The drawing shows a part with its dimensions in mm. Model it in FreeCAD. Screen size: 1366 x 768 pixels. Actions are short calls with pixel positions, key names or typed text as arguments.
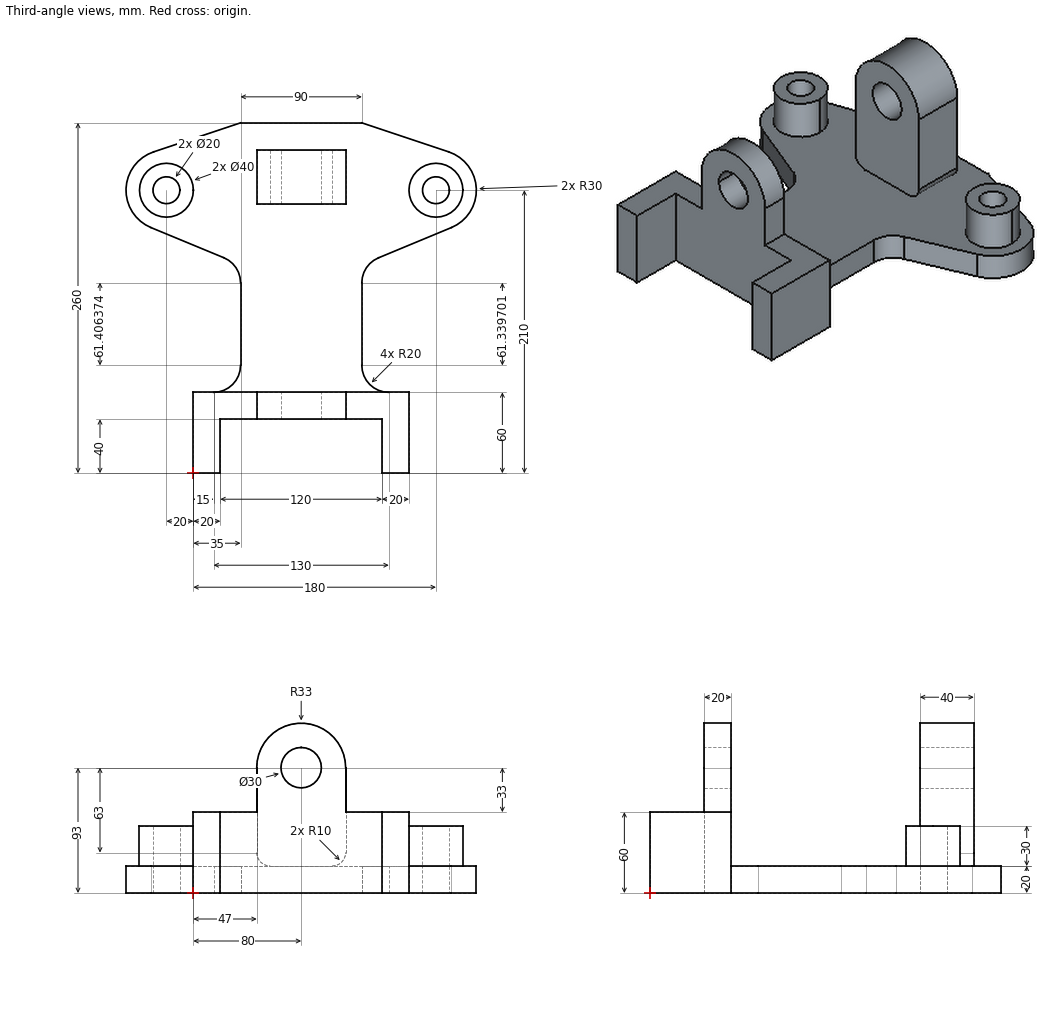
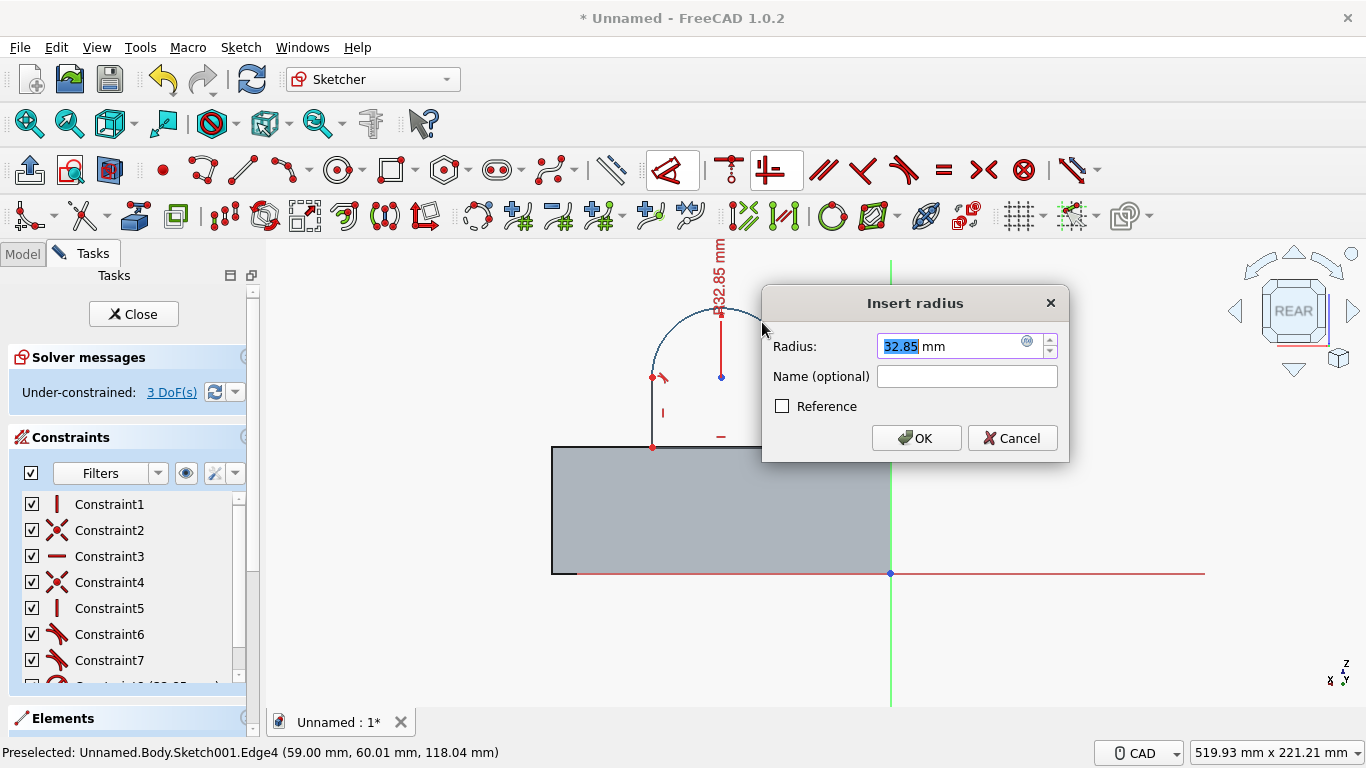
text(33)
key(Return)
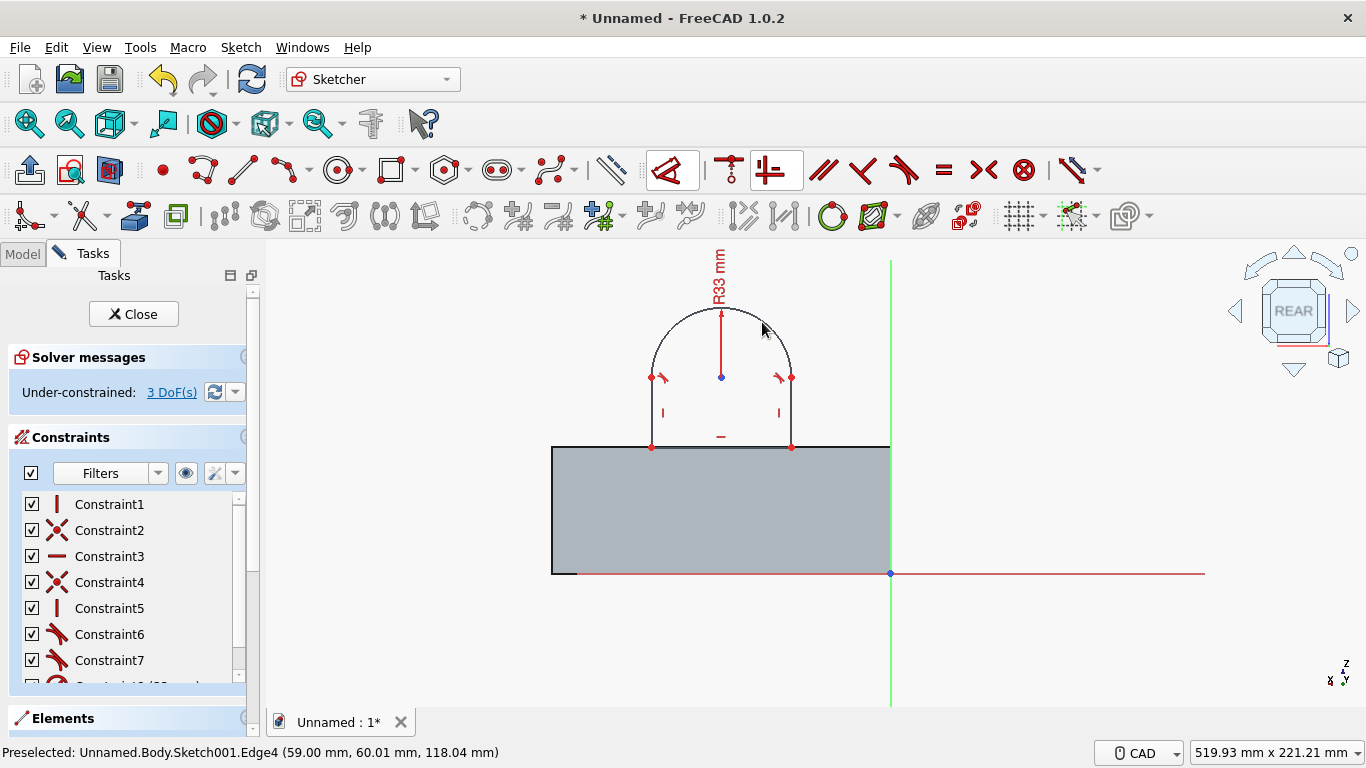
click(652, 399)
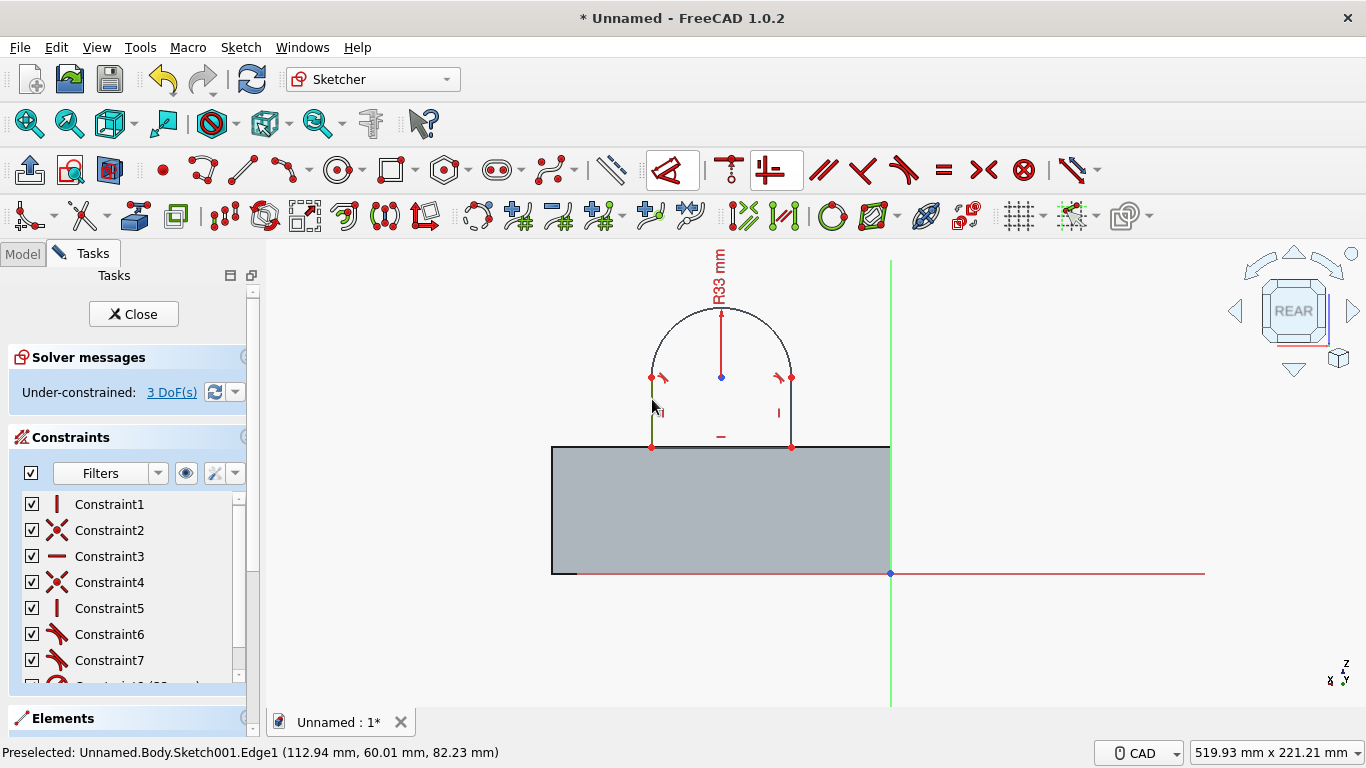
click(694, 170)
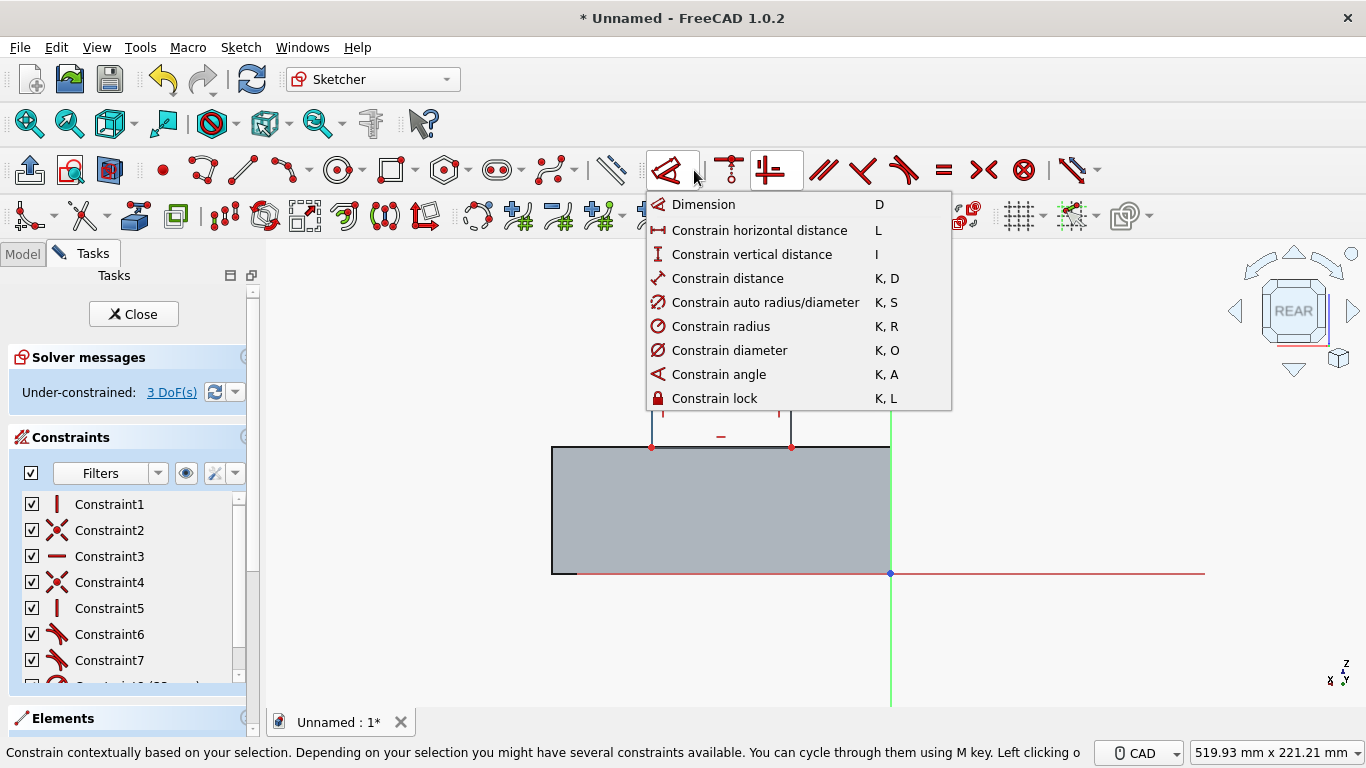
click(799, 254)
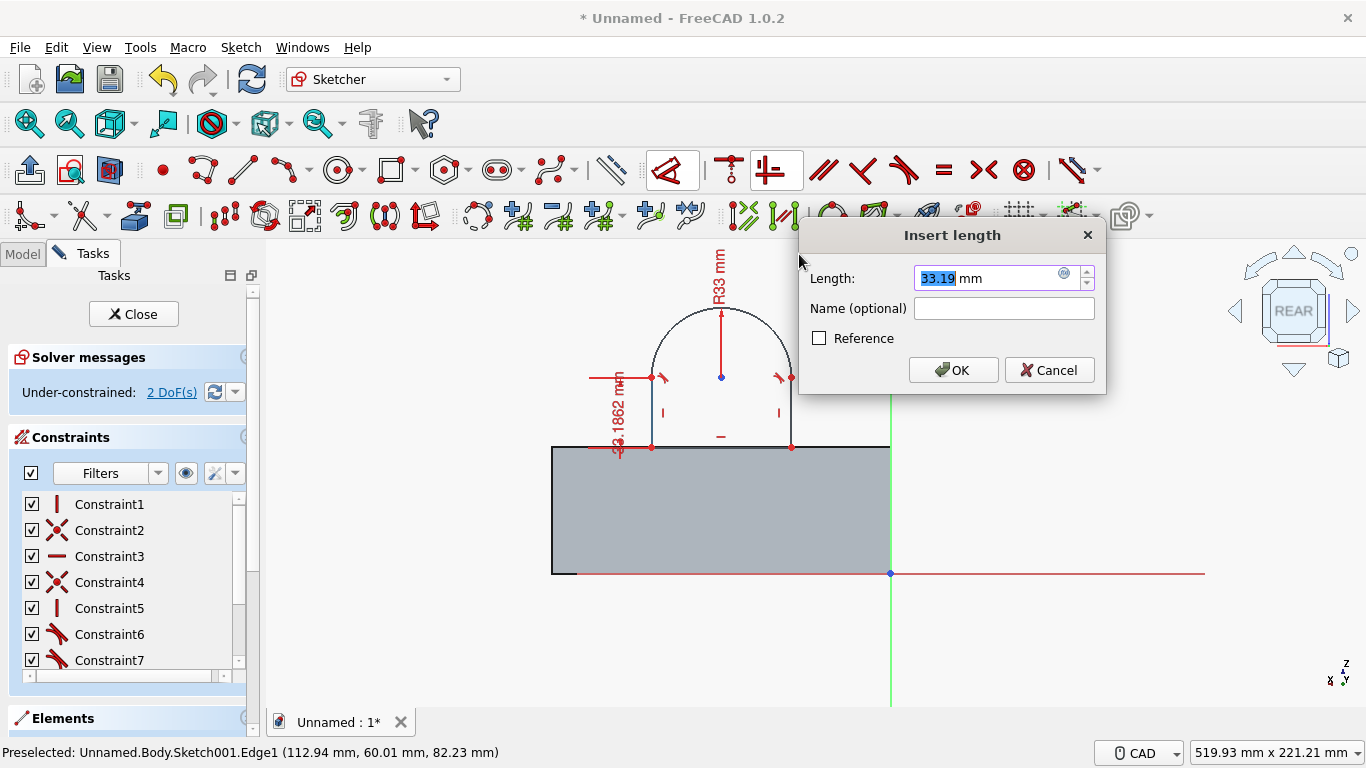
text(33)
key(Return)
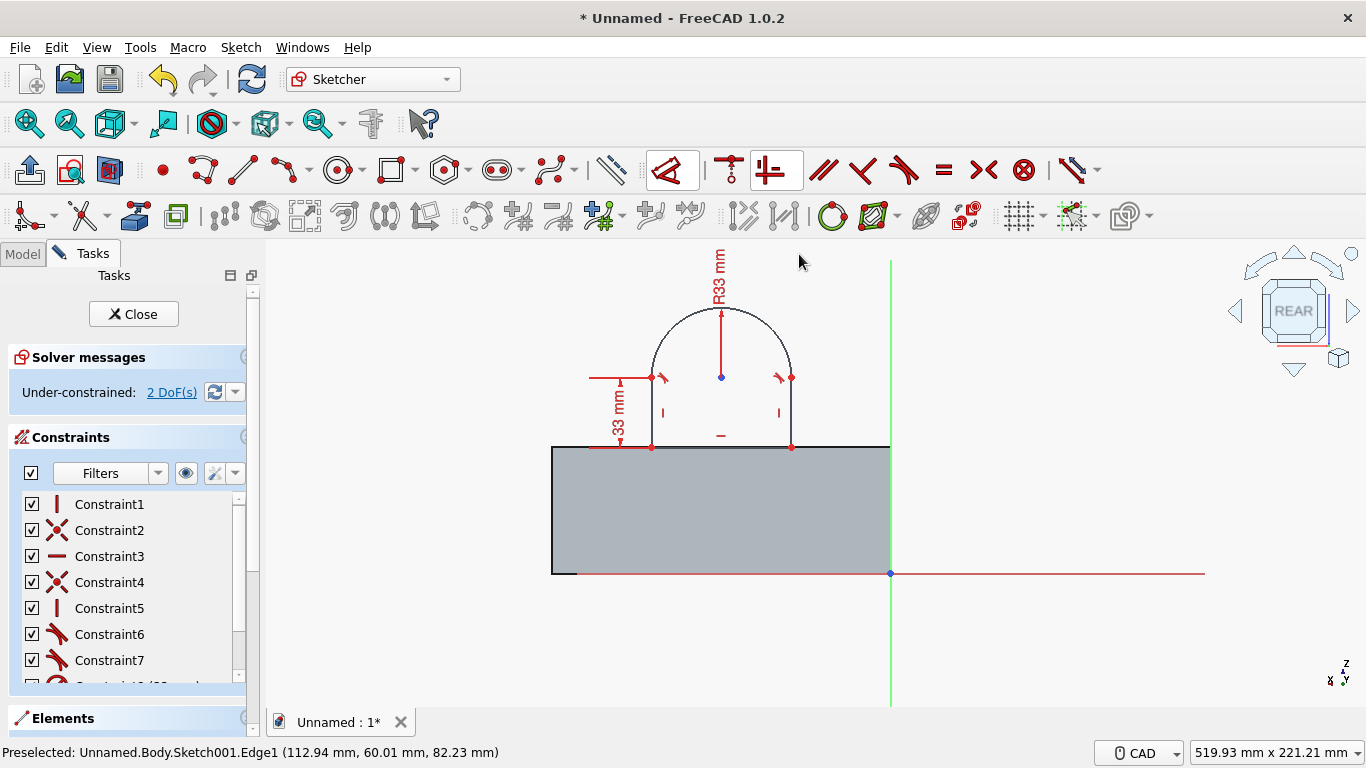
click(652, 378)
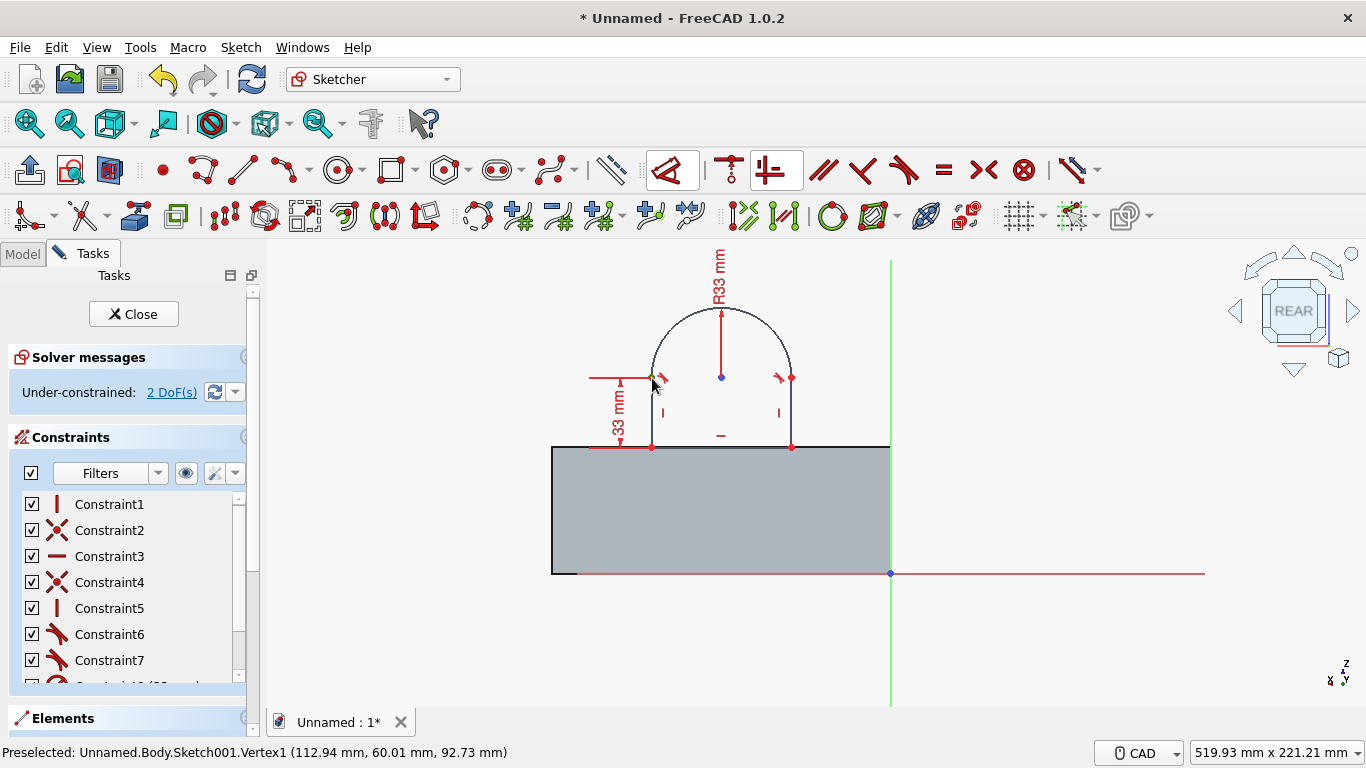
key(i)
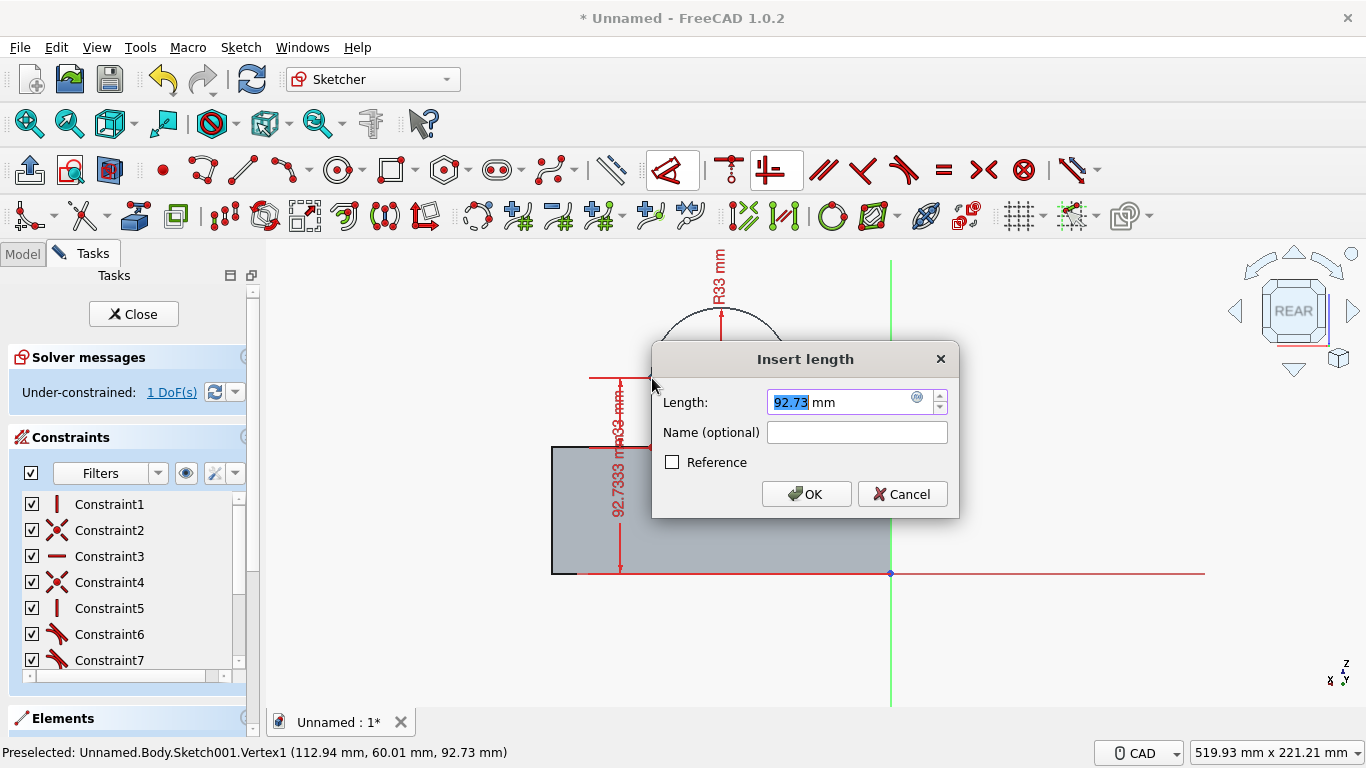
text(93)
key(Return)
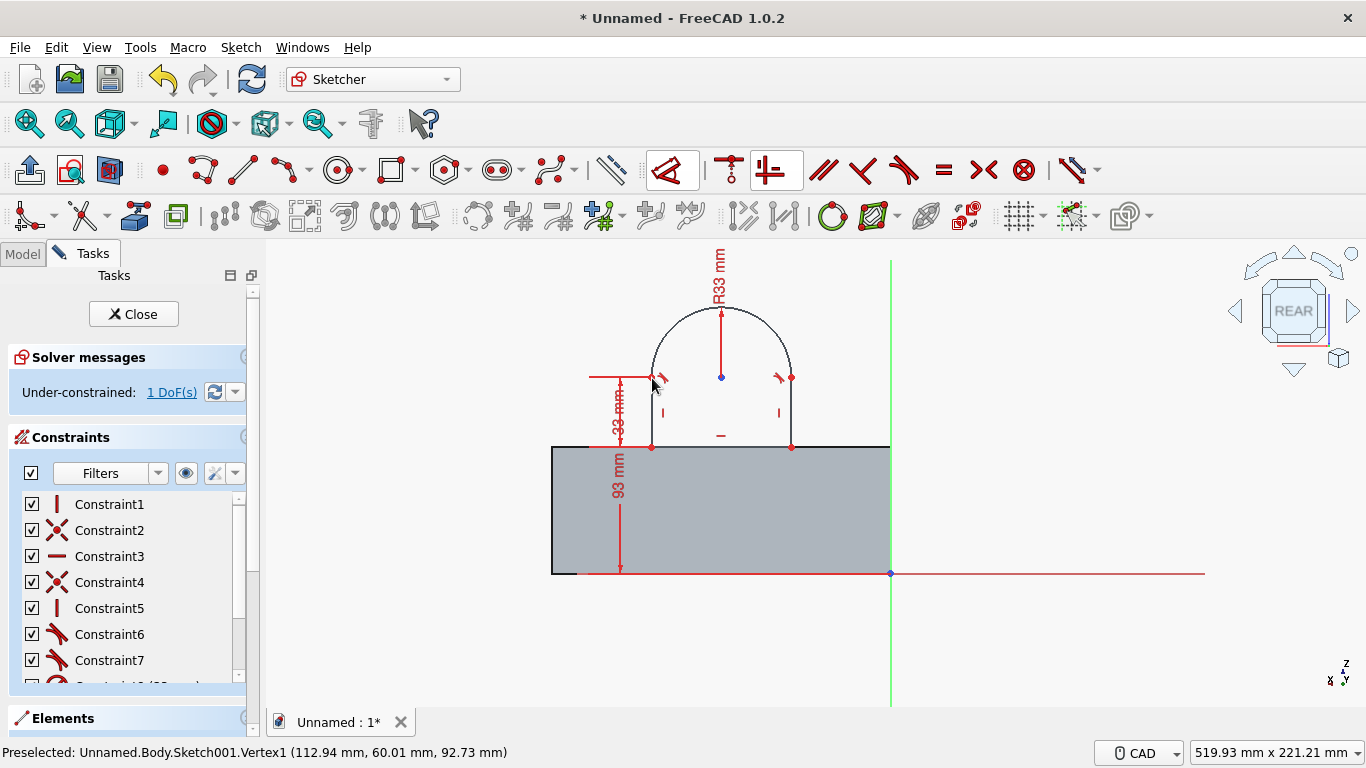
click(791, 447)